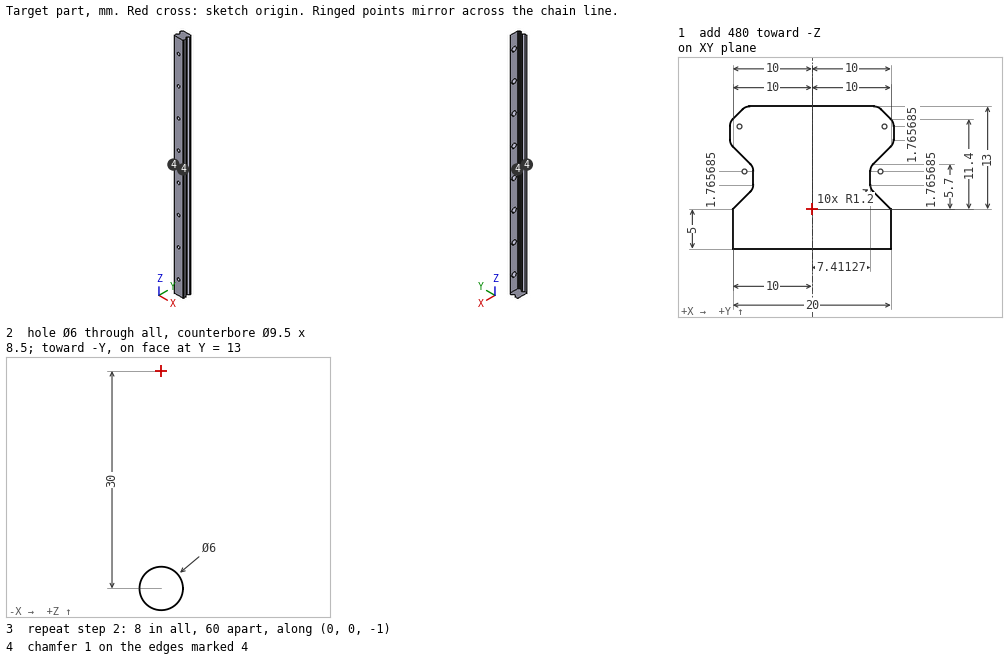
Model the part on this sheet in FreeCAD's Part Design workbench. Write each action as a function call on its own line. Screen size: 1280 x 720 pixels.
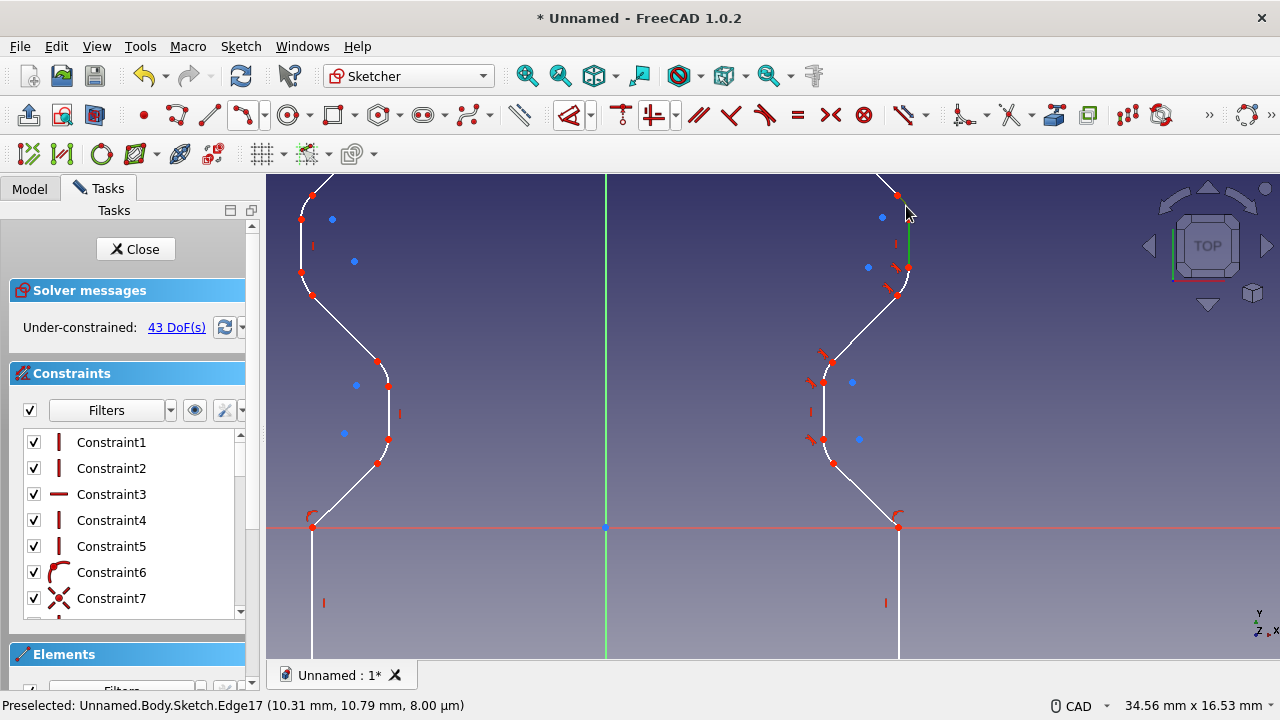
key(t)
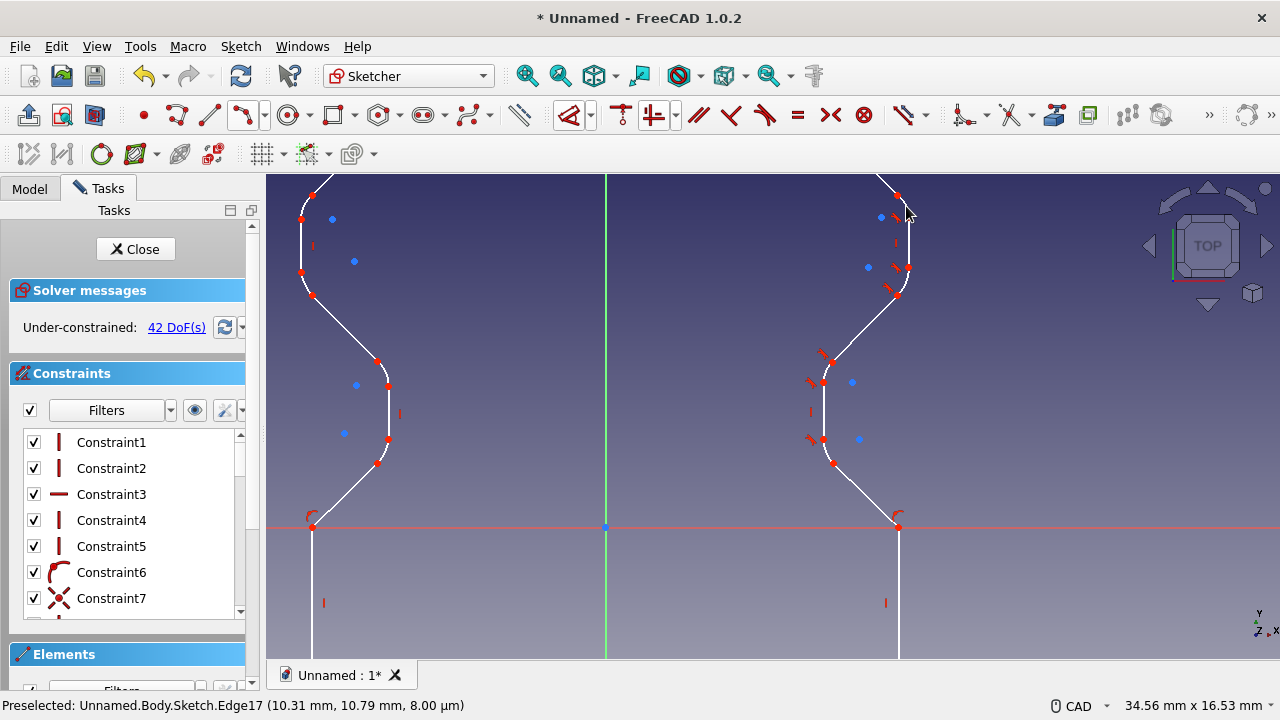
scroll(825, 424, down, 3)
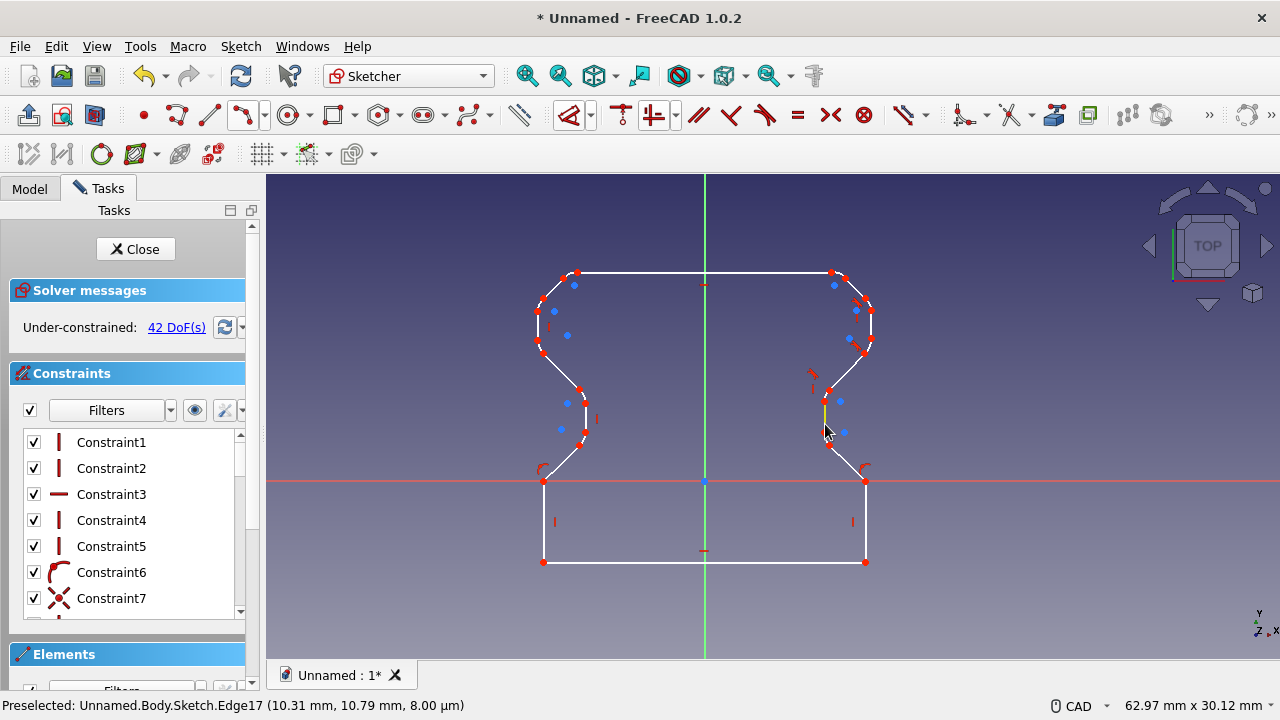
scroll(859, 293, up, 3)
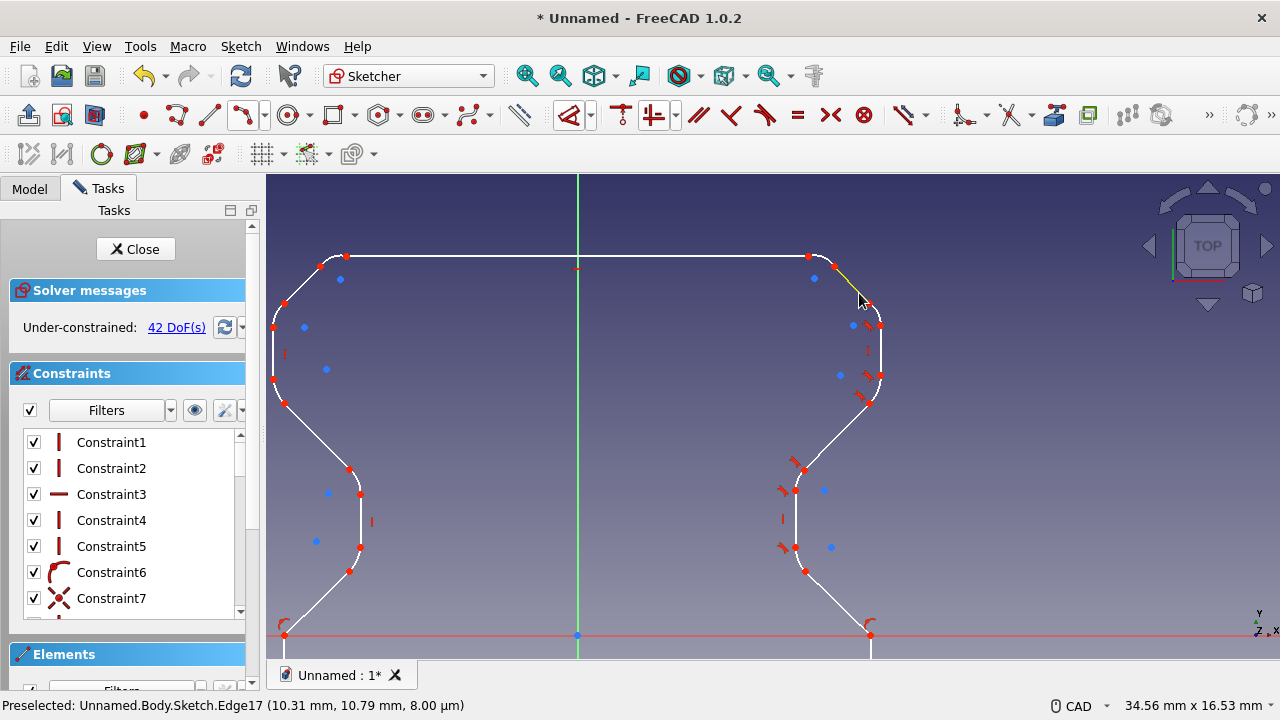
click(859, 292)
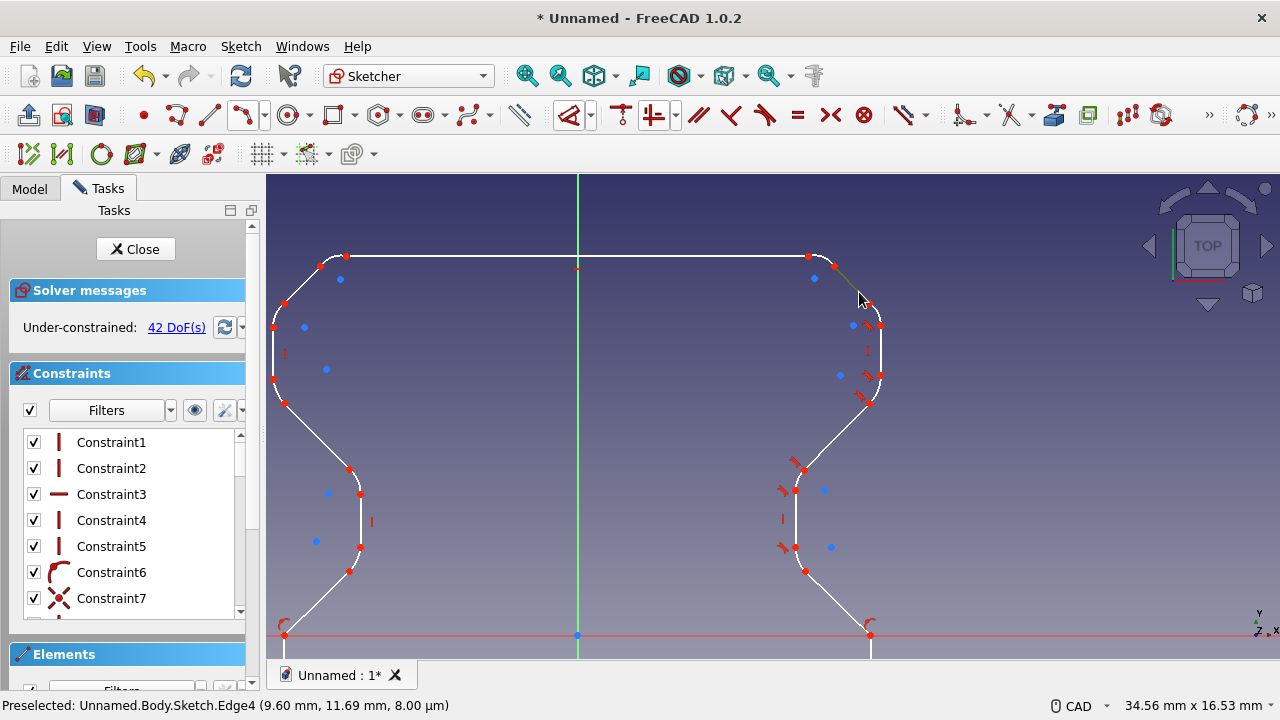
click(878, 313)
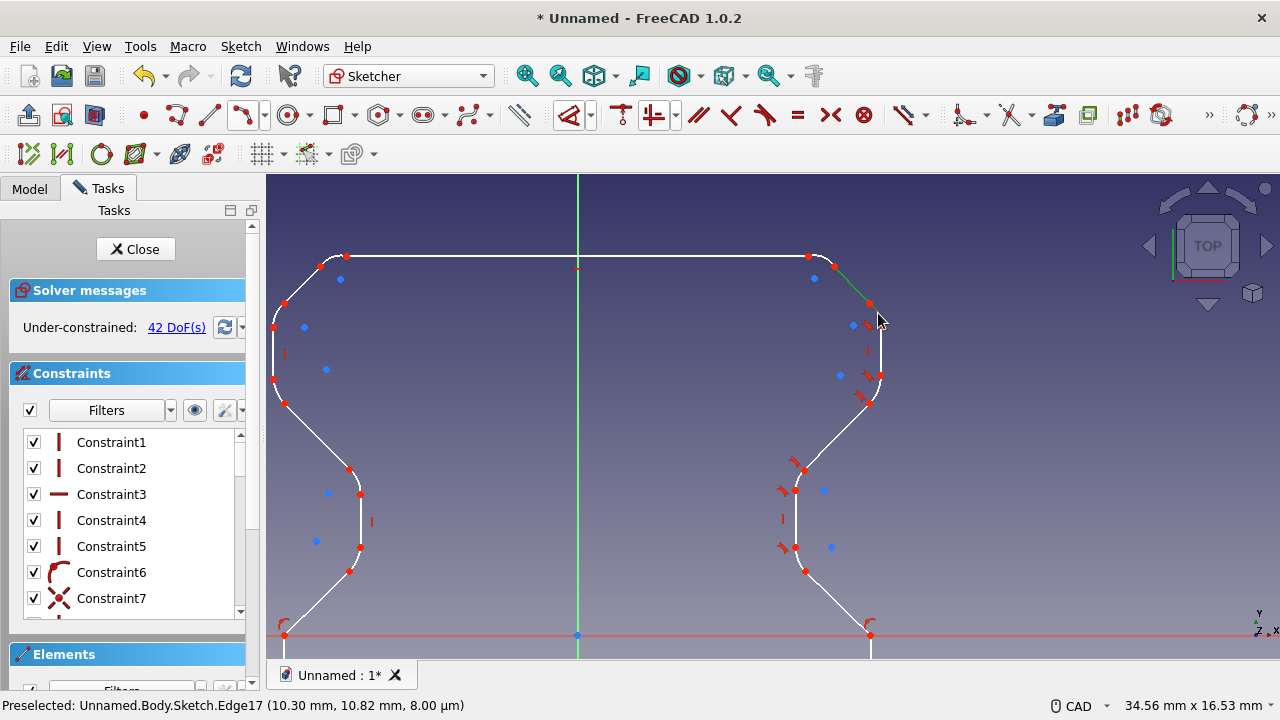
key(t)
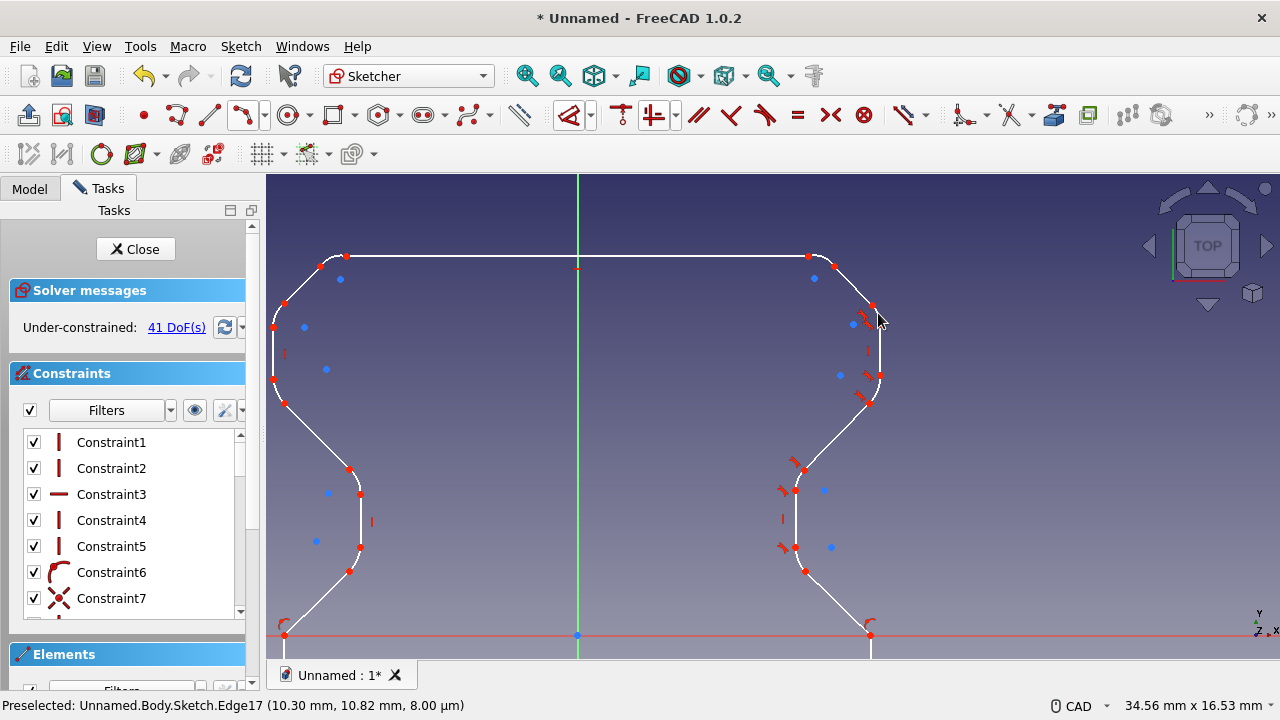
click(861, 294)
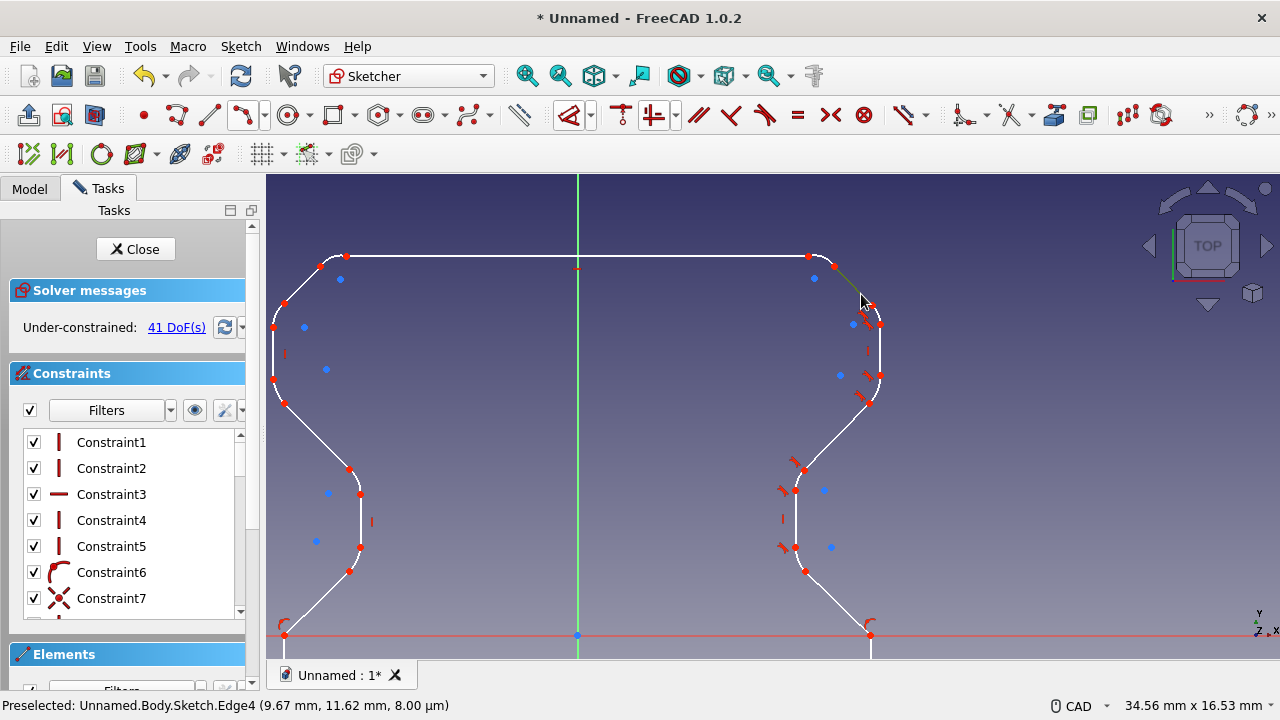
click(823, 257)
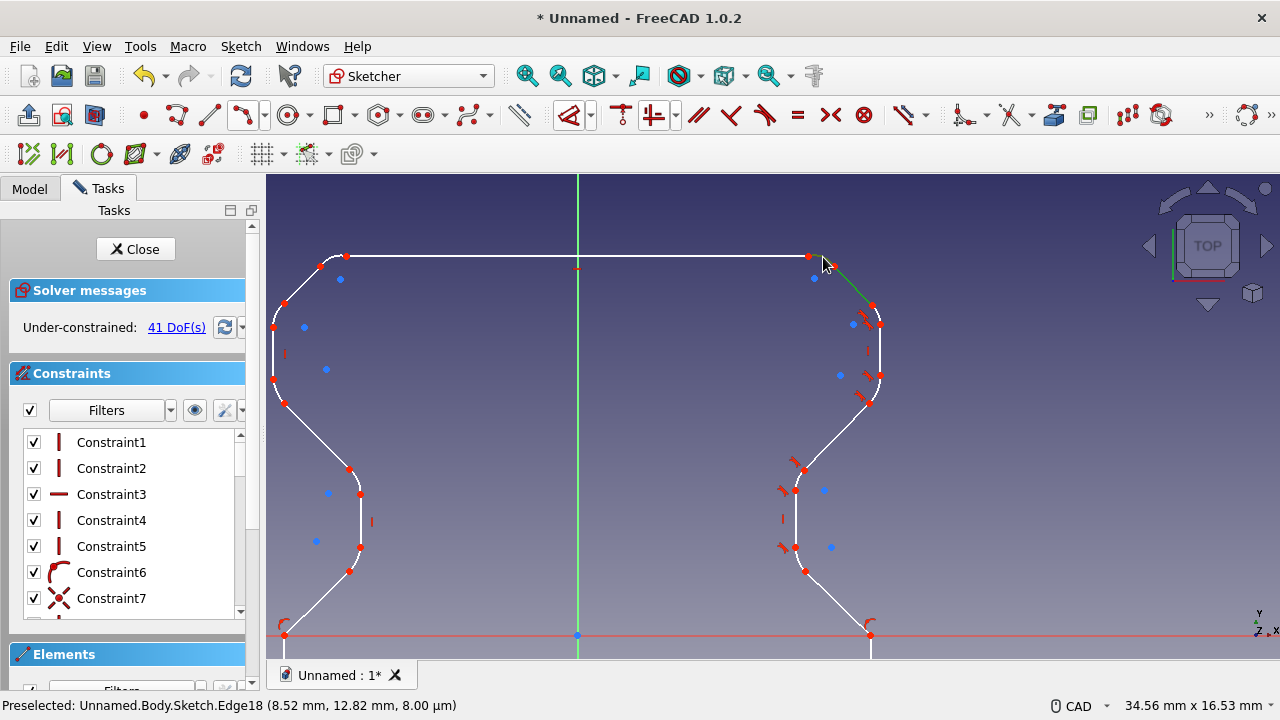
key(t)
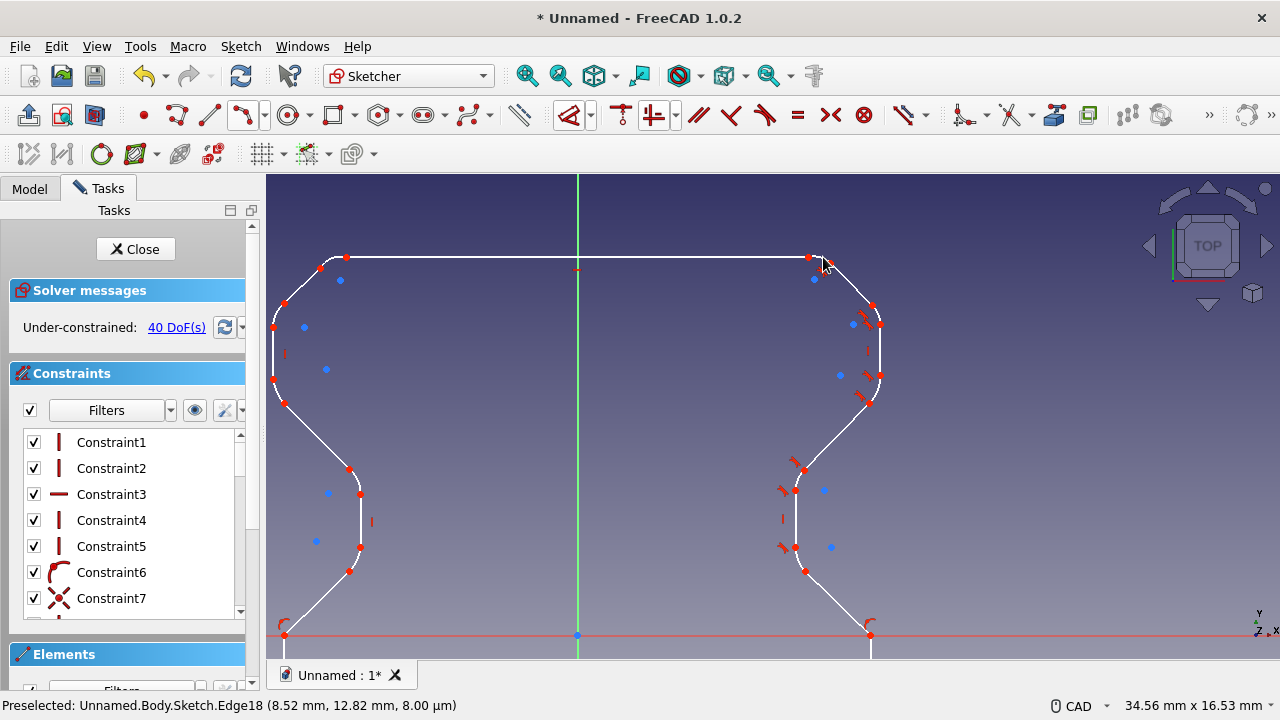
click(670, 257)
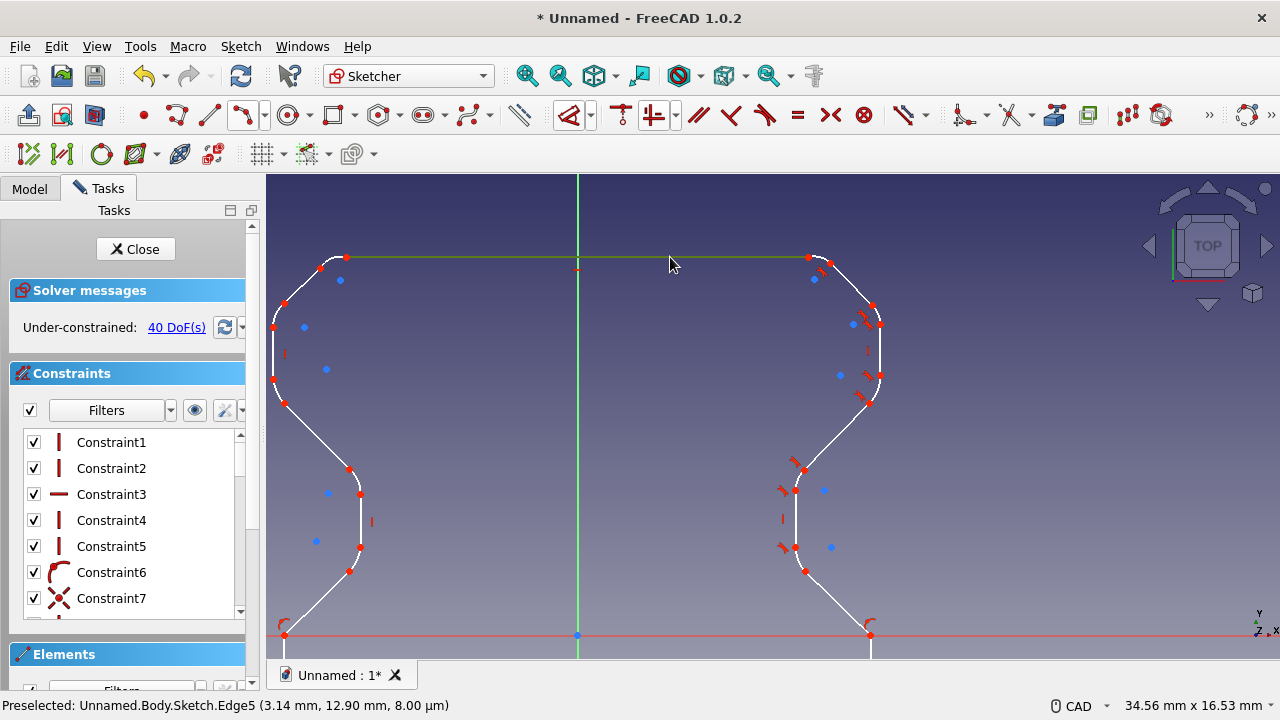
click(821, 257)